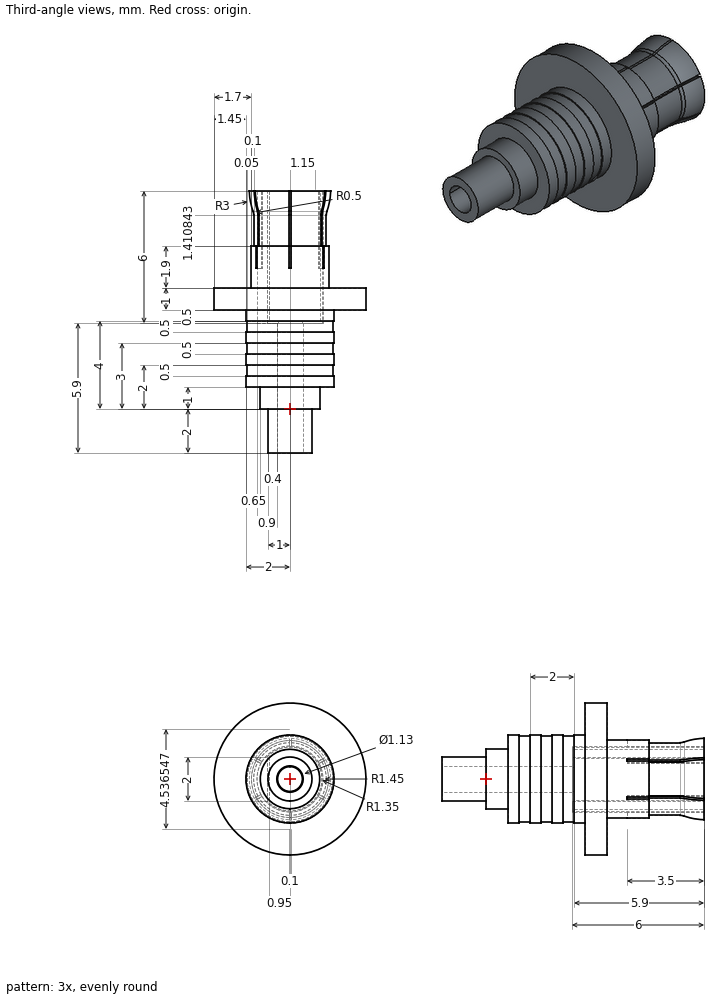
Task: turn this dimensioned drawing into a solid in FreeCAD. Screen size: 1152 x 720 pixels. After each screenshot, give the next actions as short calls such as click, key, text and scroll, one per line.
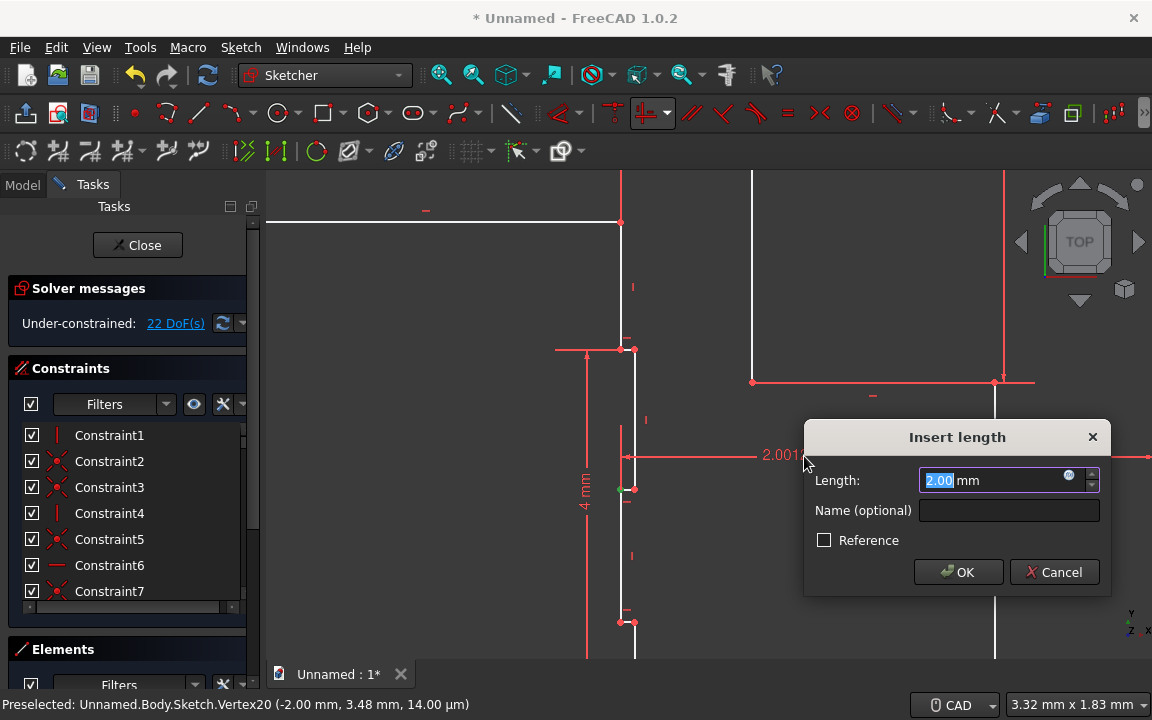
text(2)
key(Return)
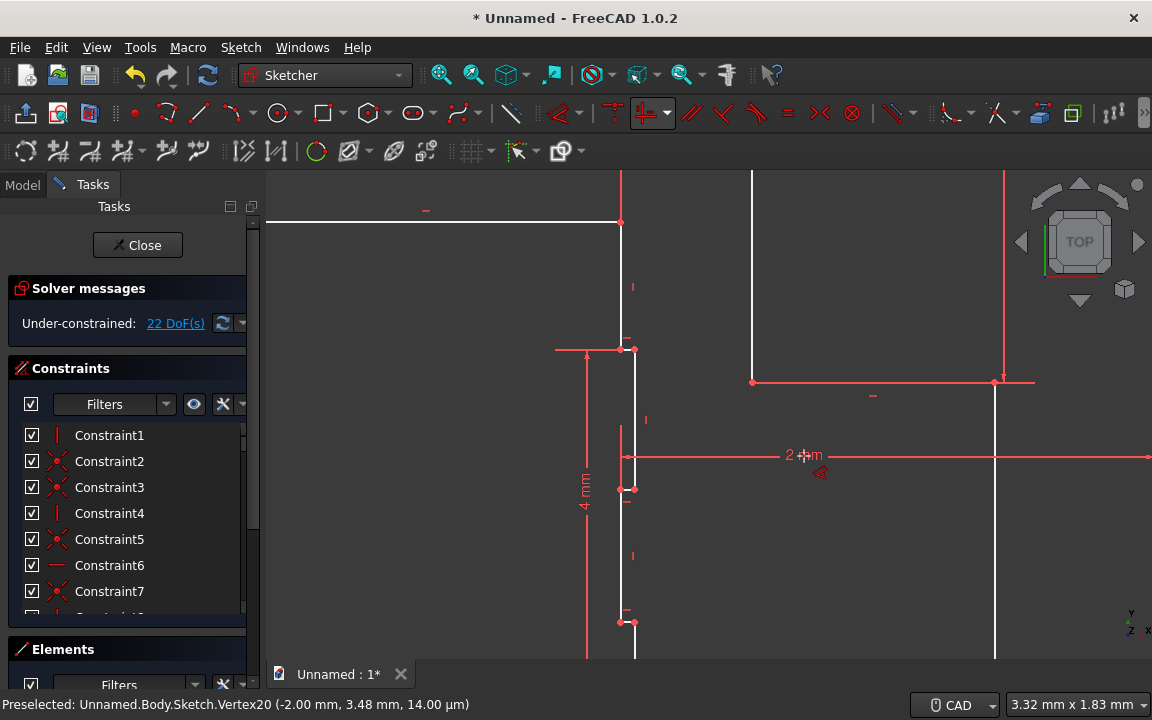
click(621, 622)
click(587, 627)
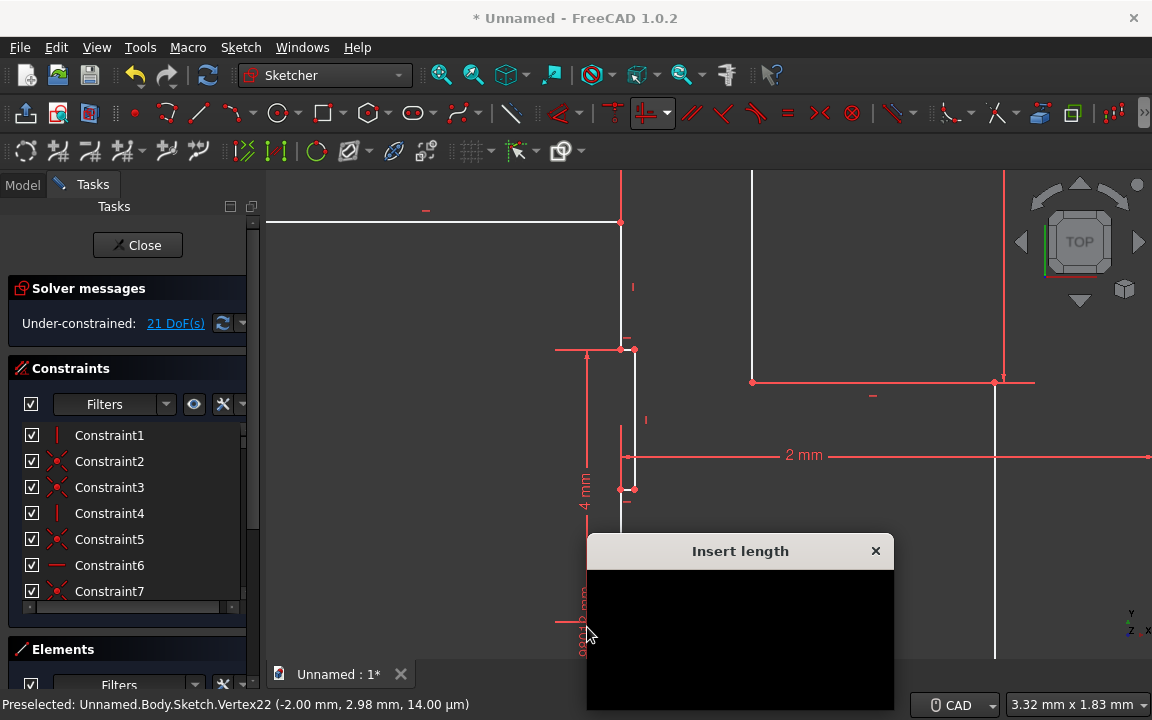
text(3)
key(Return)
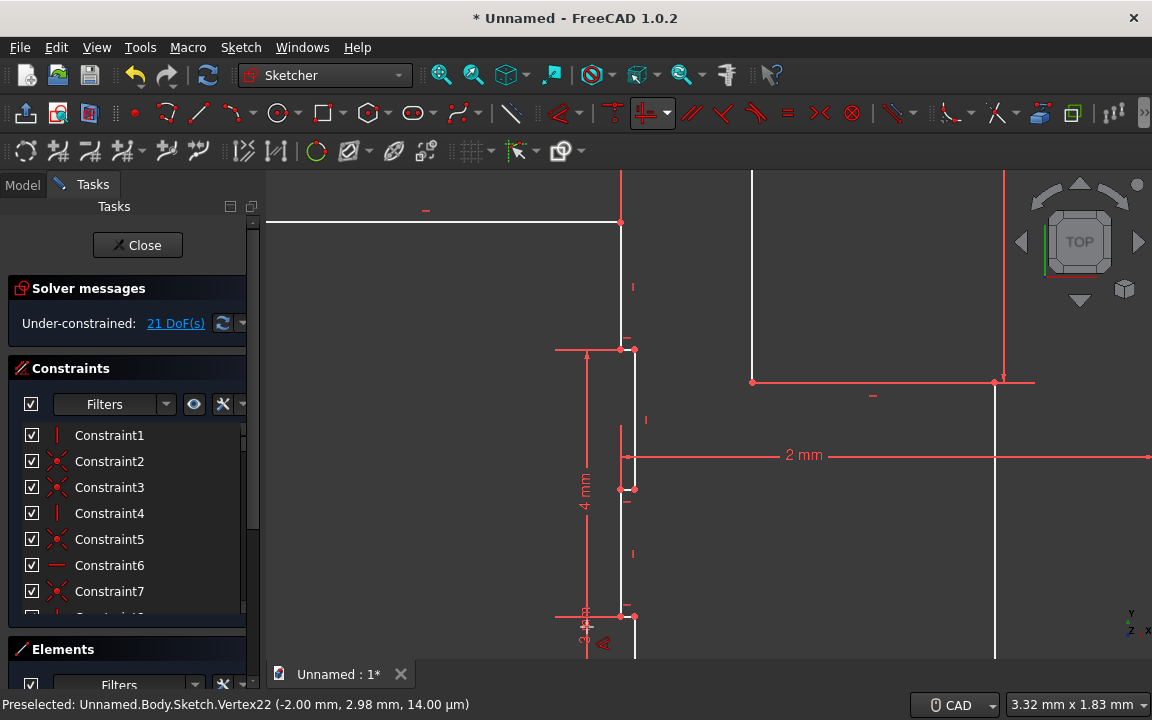
scroll(635, 420, down, 12)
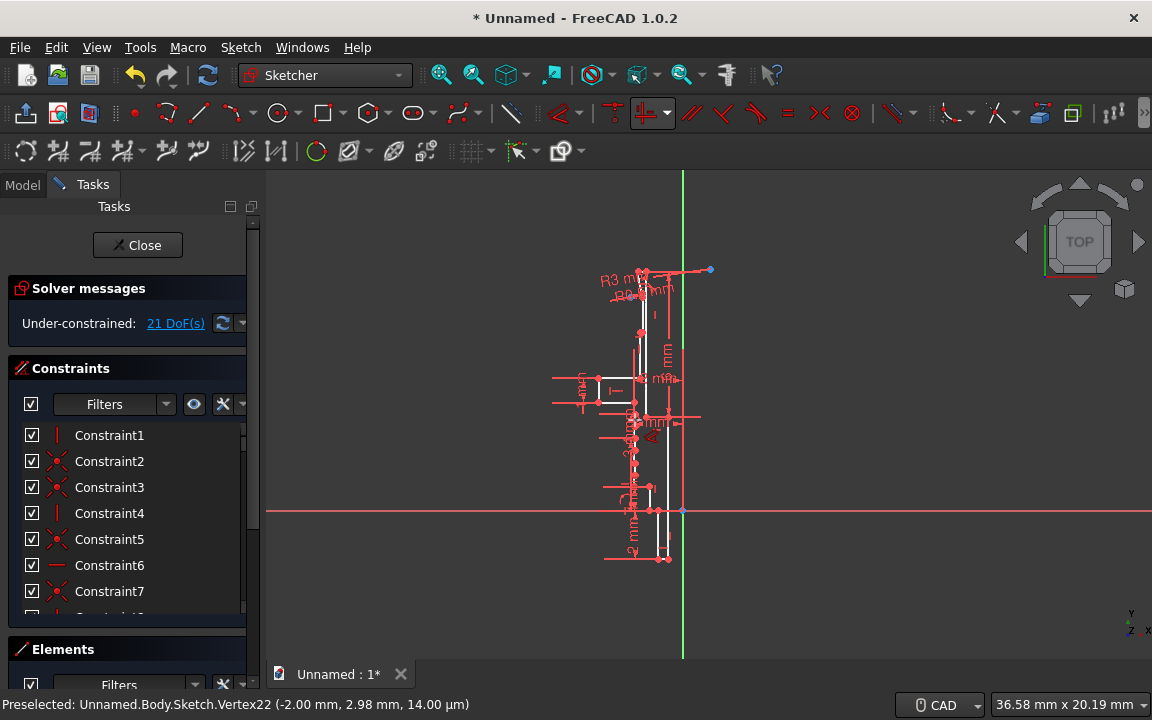
scroll(634, 451, up, 12)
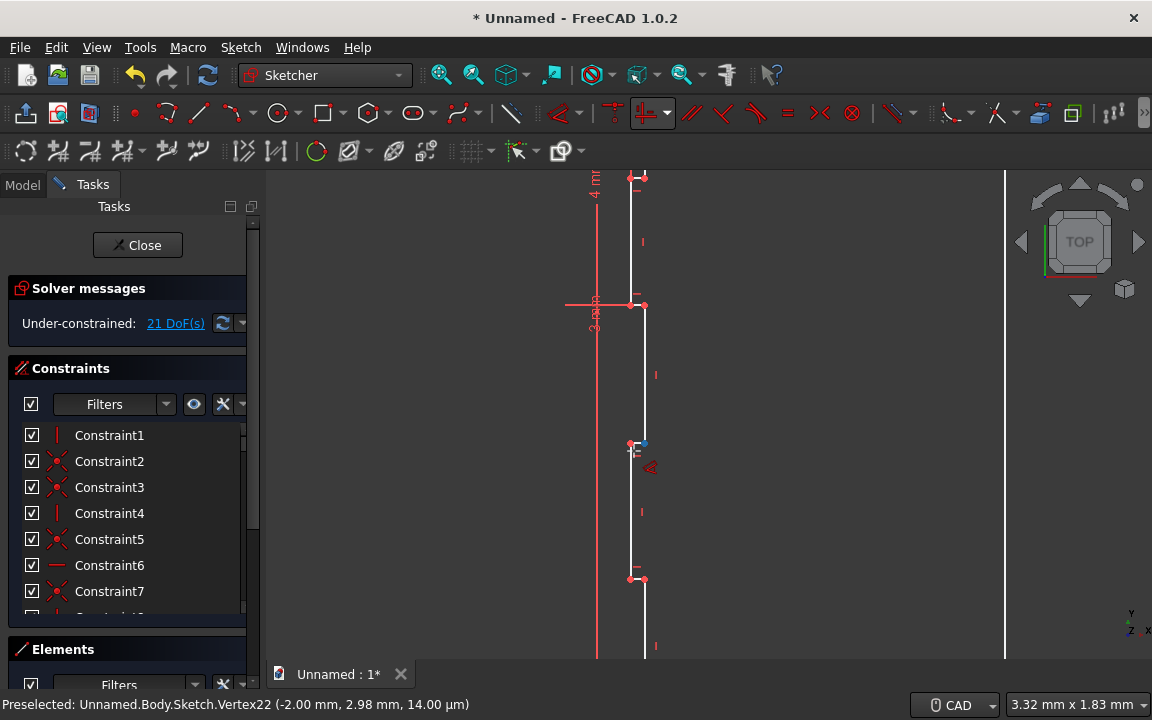
click(631, 443)
click(809, 409)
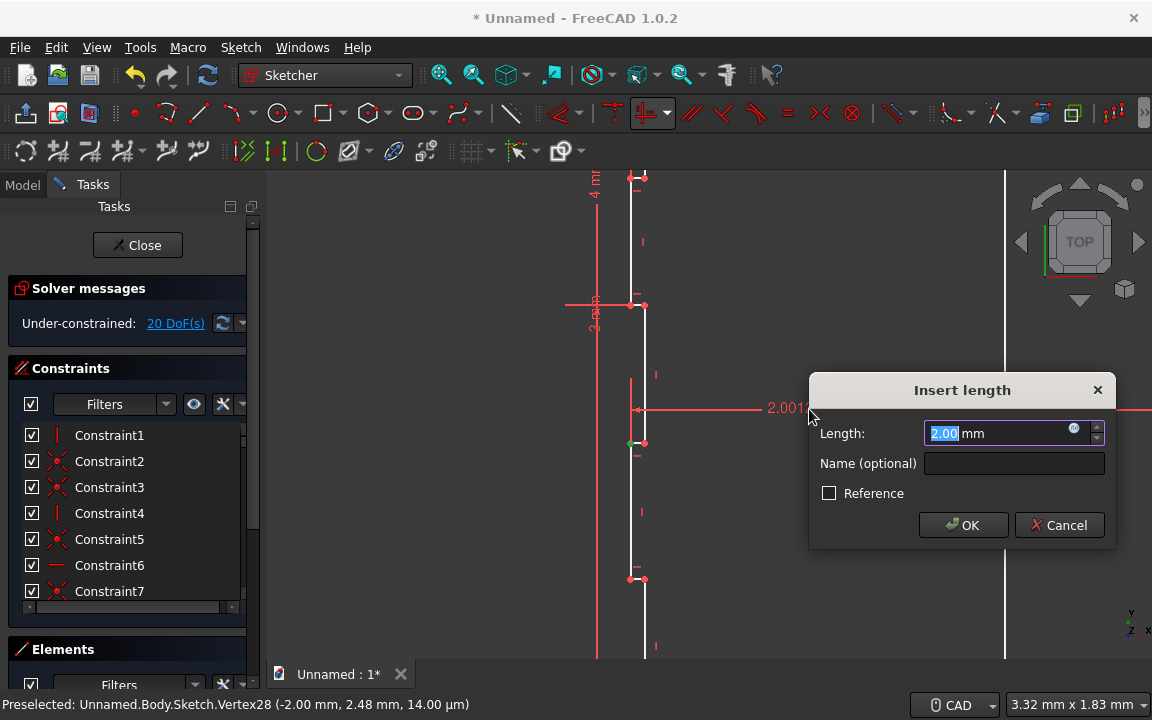
text(2)
key(Return)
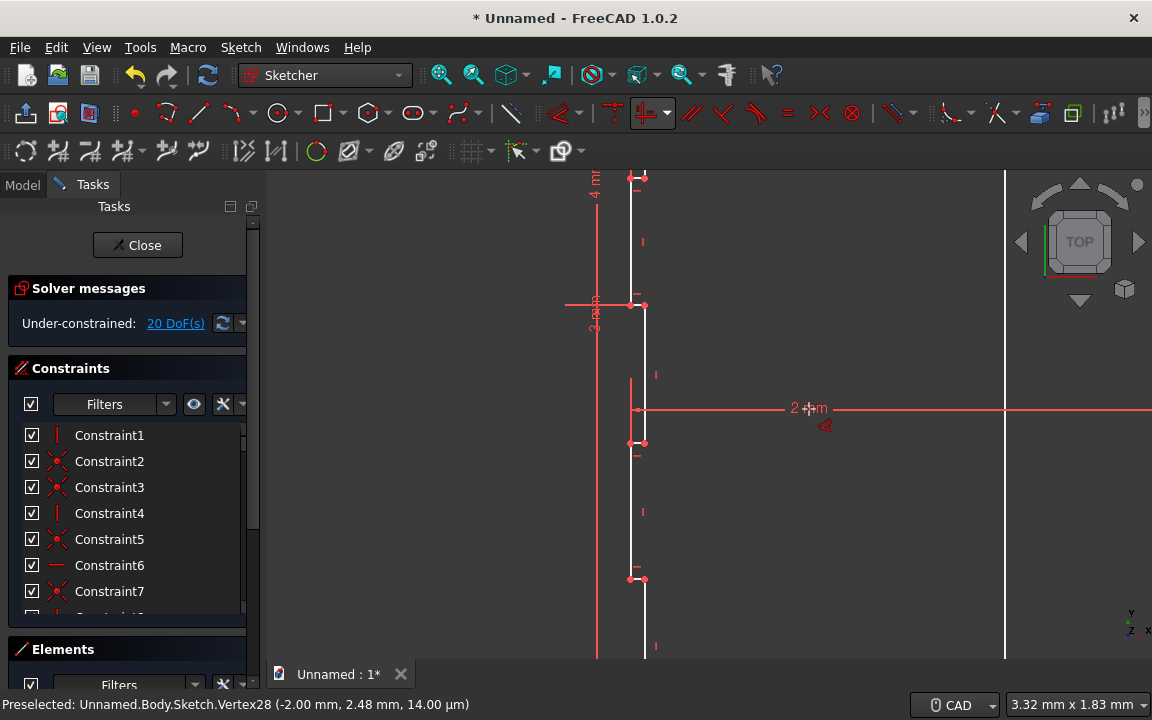
click(631, 579)
click(597, 605)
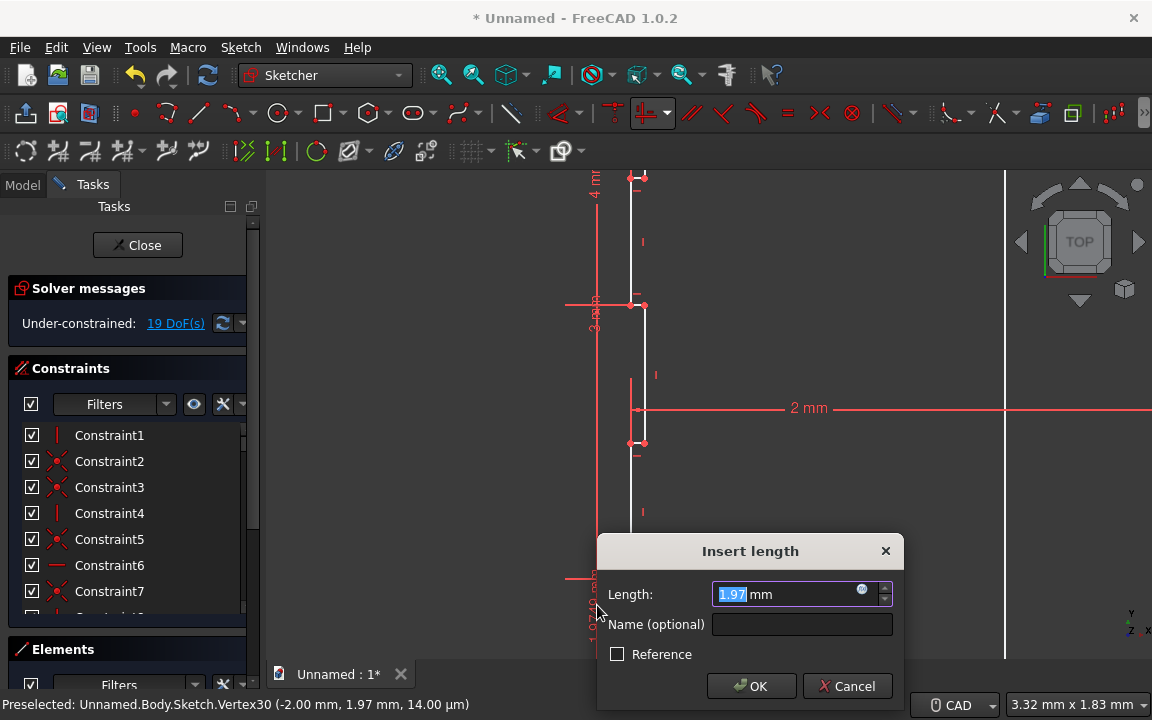
text(2)
key(Return)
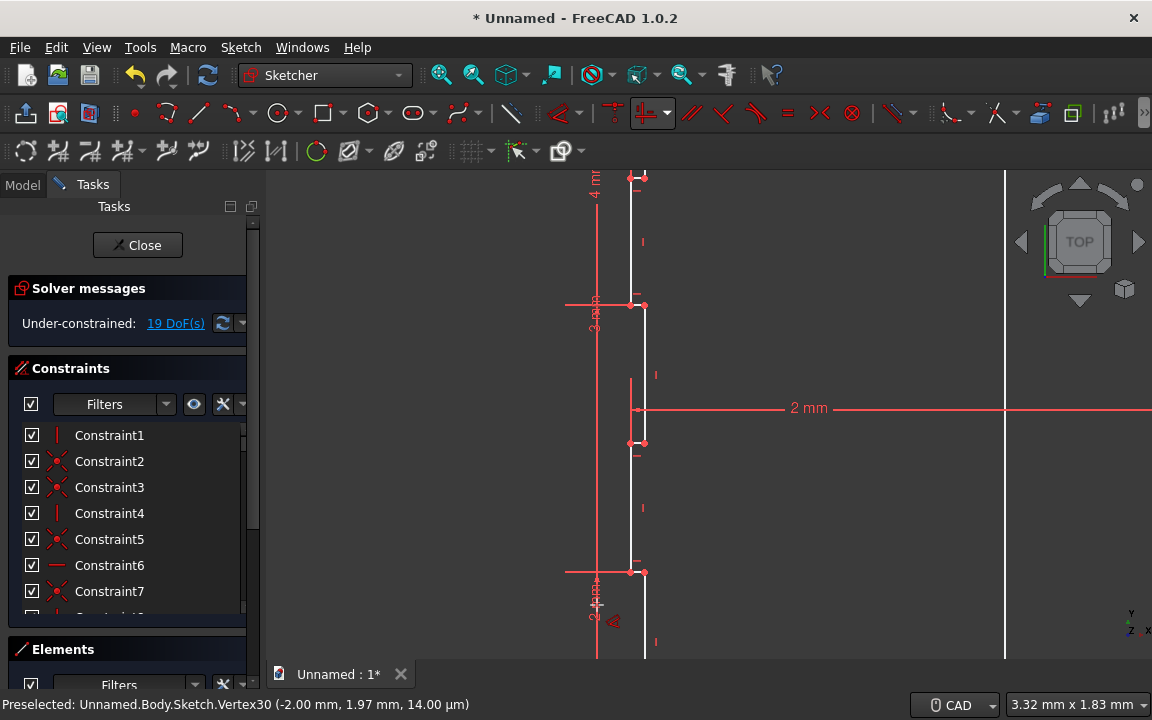
scroll(634, 451, down, 12)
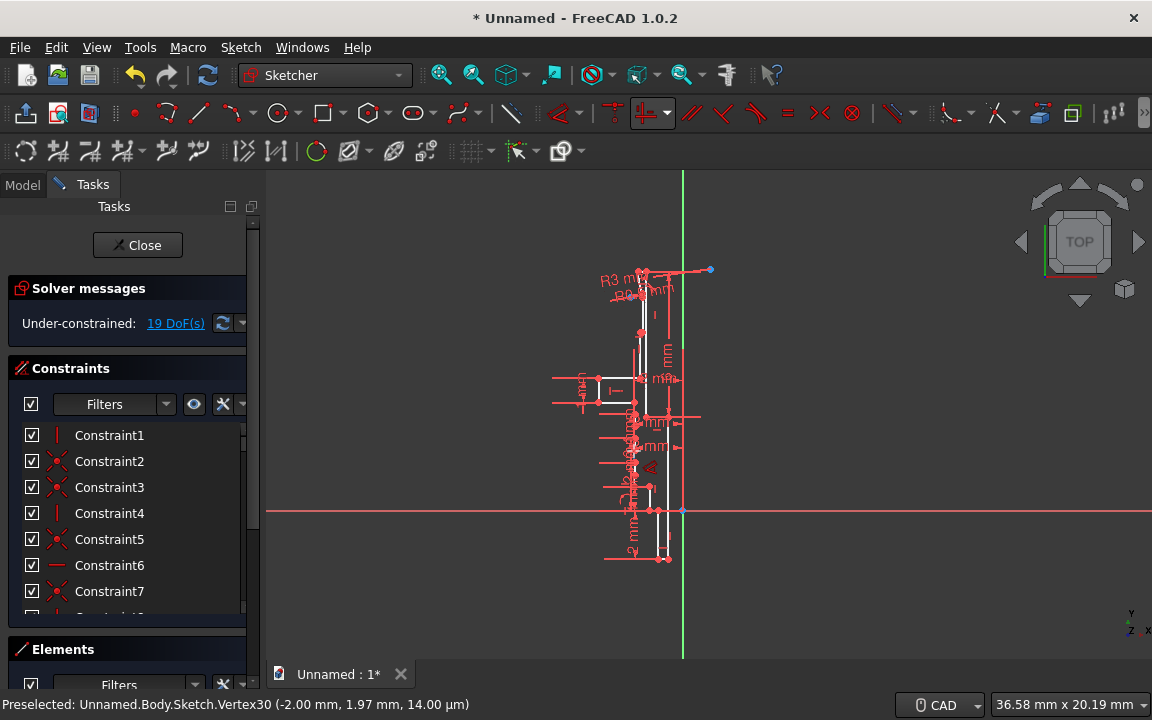
scroll(634, 475, up, 12)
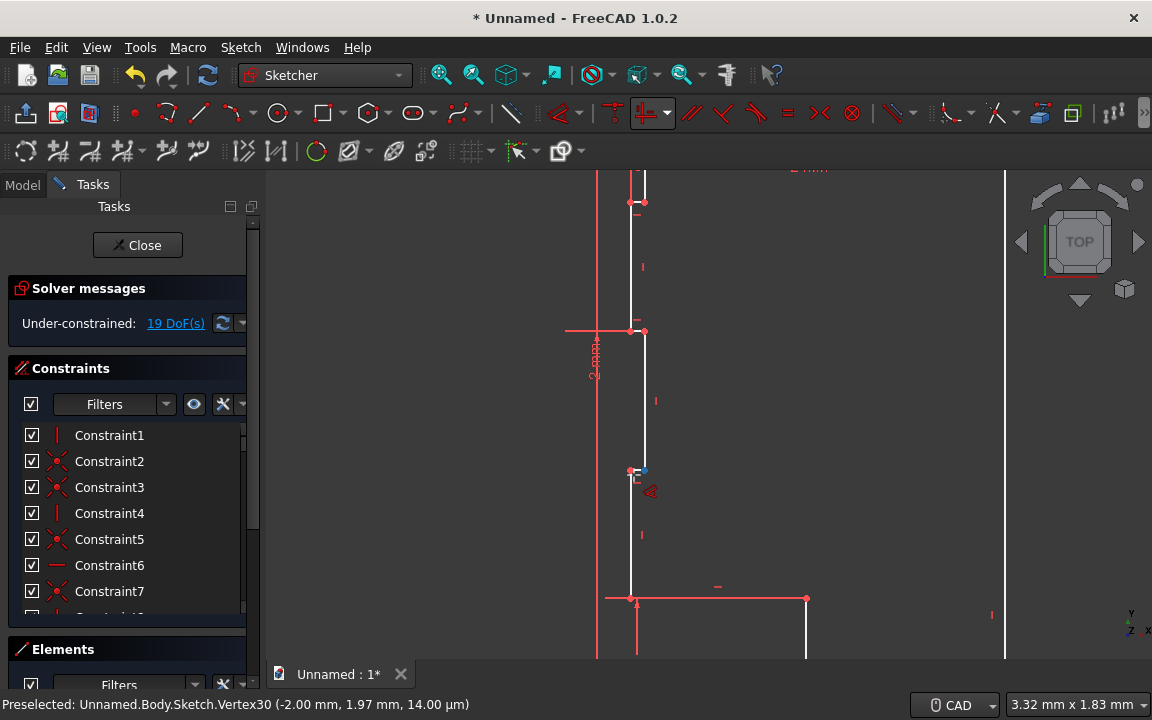
click(631, 470)
click(809, 436)